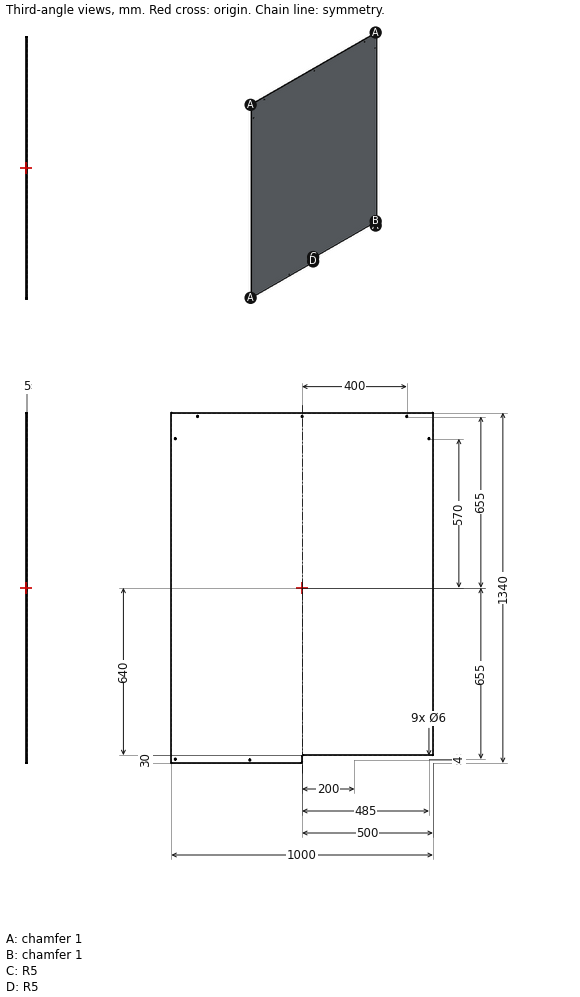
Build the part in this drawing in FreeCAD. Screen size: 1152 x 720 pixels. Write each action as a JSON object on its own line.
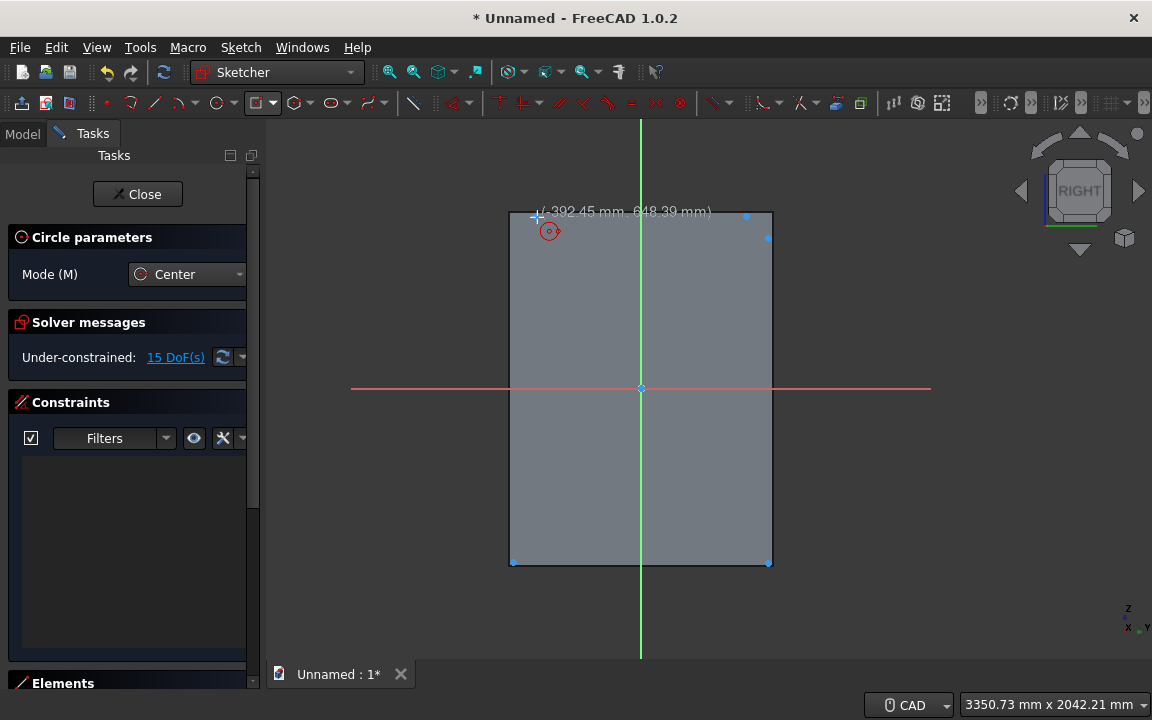
{"action": "scroll", "coordinate": [513, 238], "scroll_direction": "up", "scroll_amount": 17}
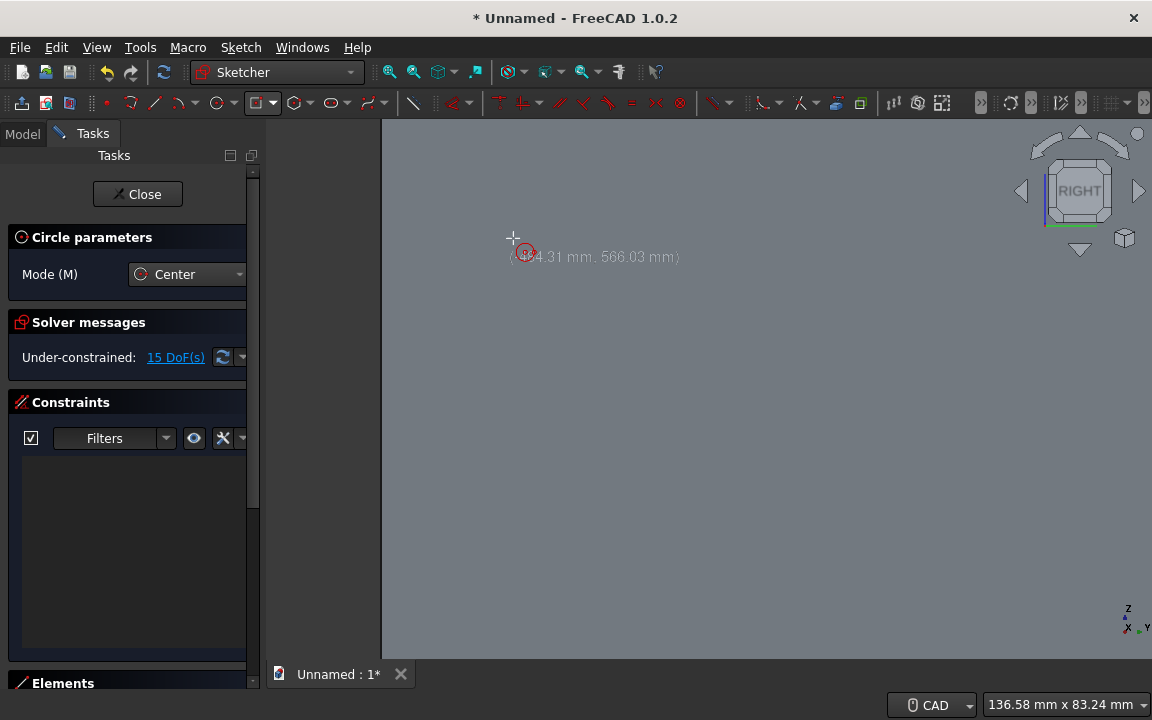
{"action": "scroll", "coordinate": [483, 203], "scroll_direction": "down", "scroll_amount": 16}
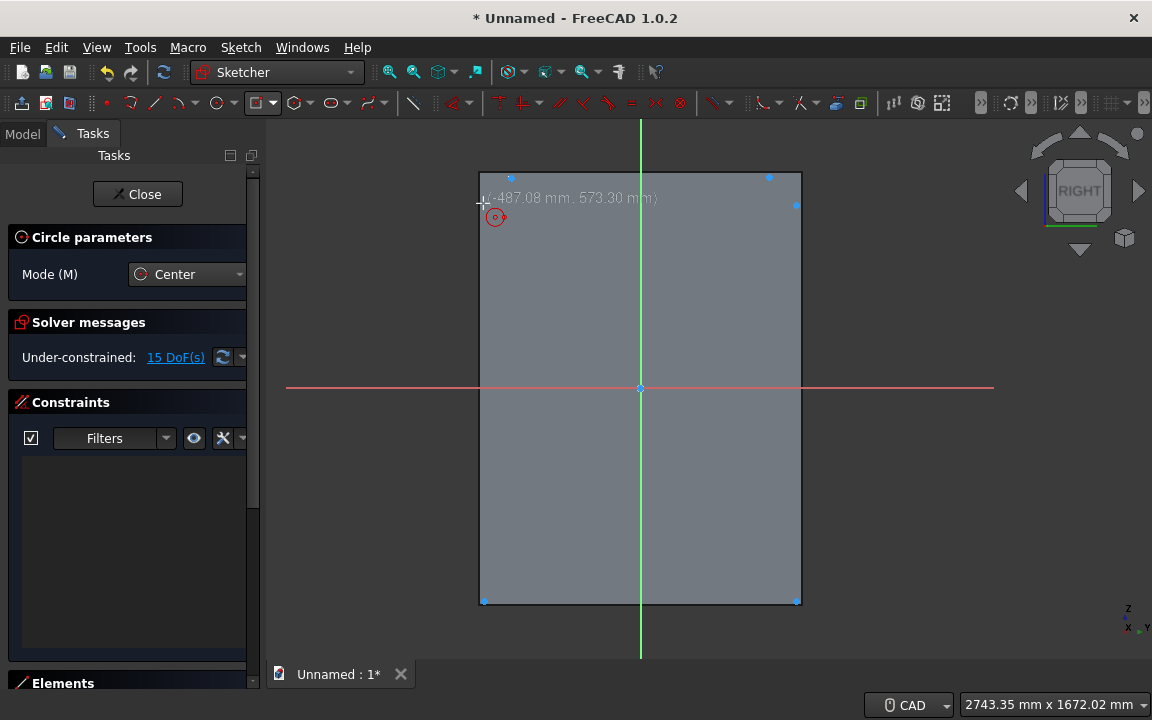
{"action": "left_click", "coordinate": [484, 204]}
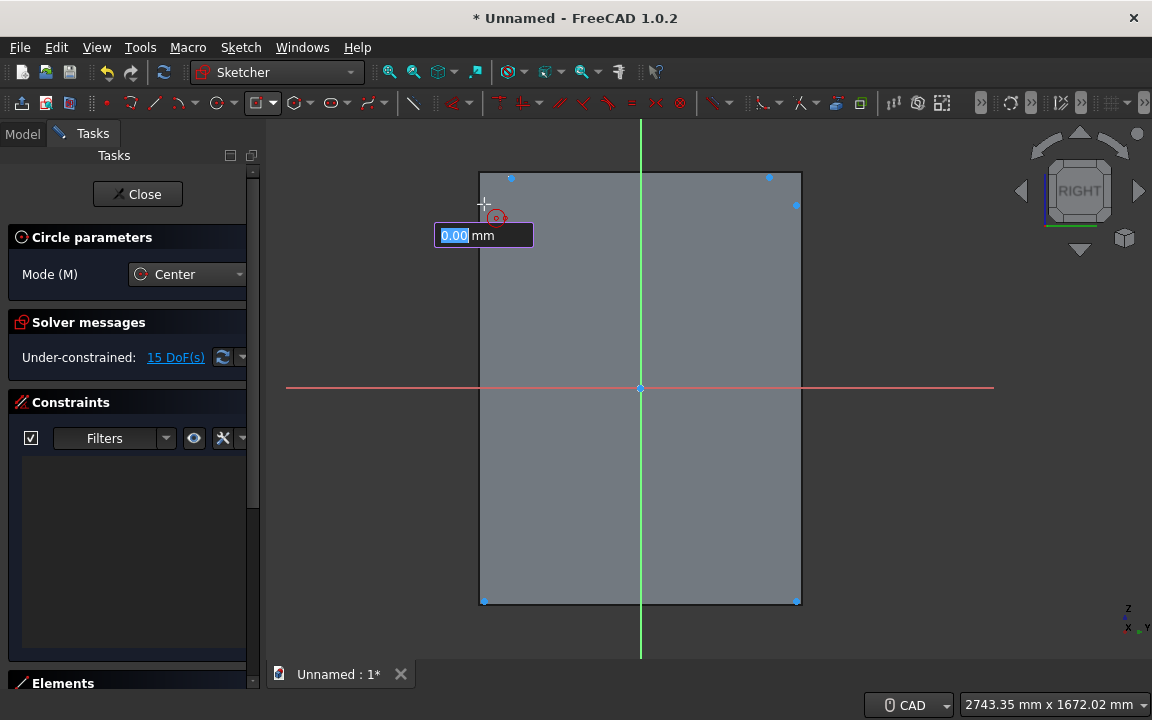
{"action": "scroll", "coordinate": [485, 204], "scroll_direction": "up", "scroll_amount": 14}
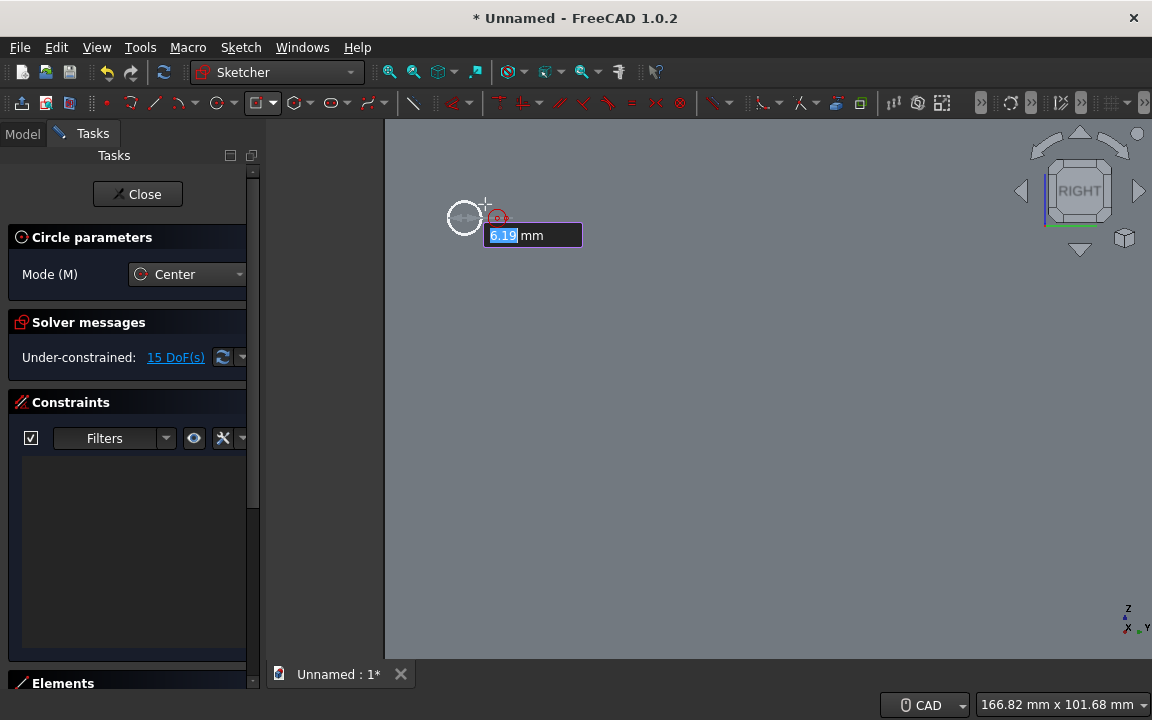
{"action": "left_click", "coordinate": [474, 194]}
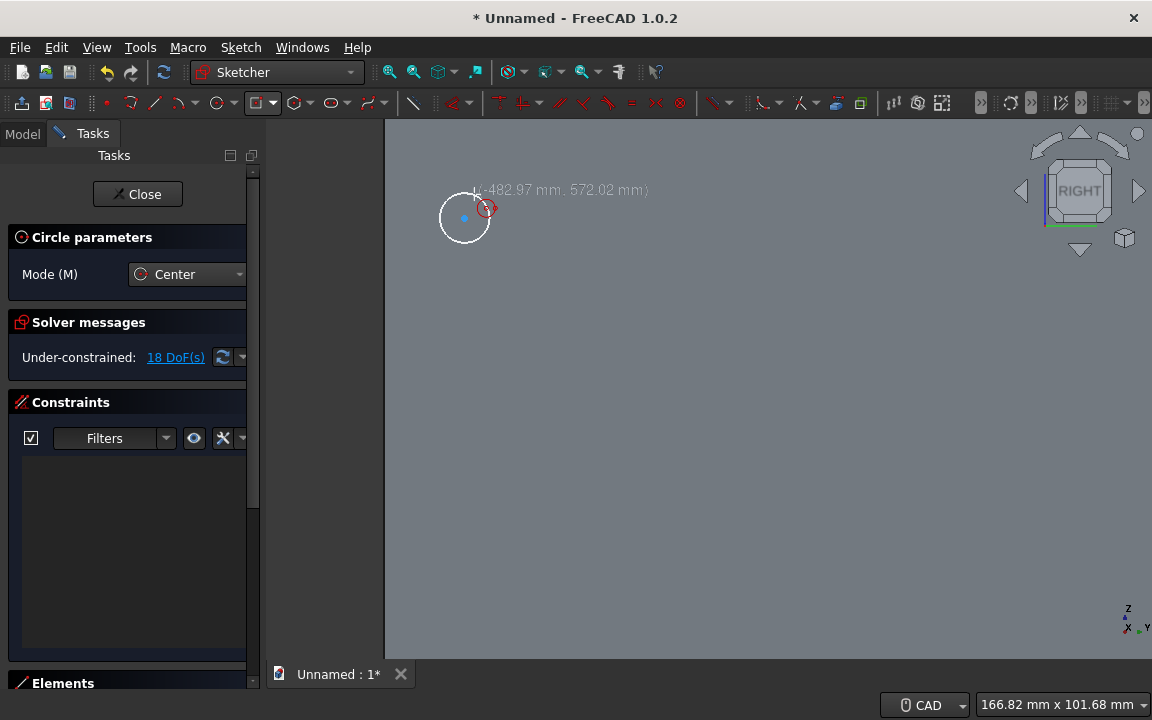
{"action": "scroll", "coordinate": [515, 239], "scroll_direction": "down", "scroll_amount": 15}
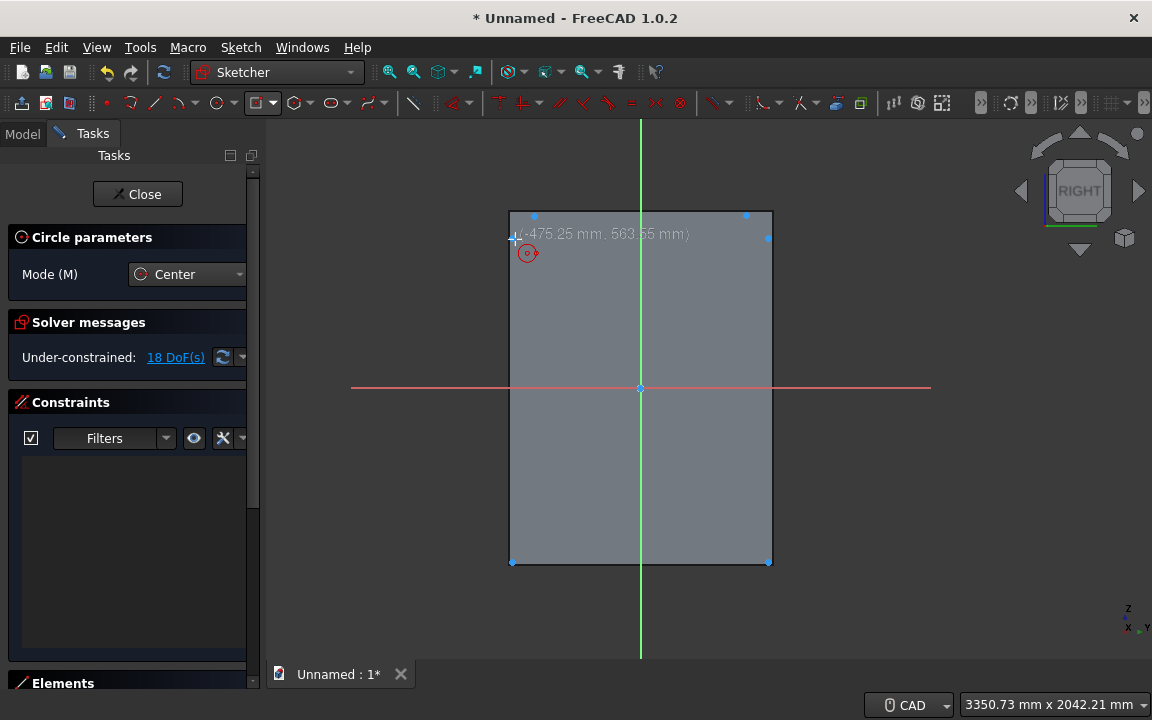
{"action": "scroll", "coordinate": [641, 215], "scroll_direction": "up", "scroll_amount": 17}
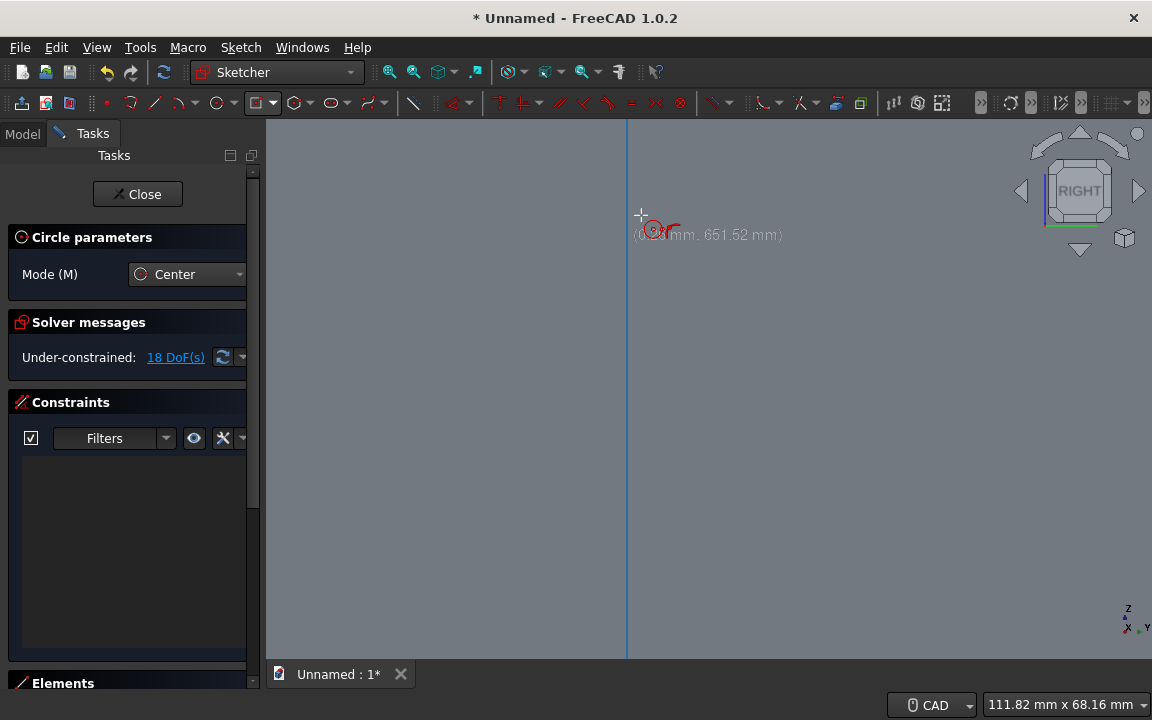
{"action": "scroll", "coordinate": [641, 175], "scroll_direction": "down", "scroll_amount": 16}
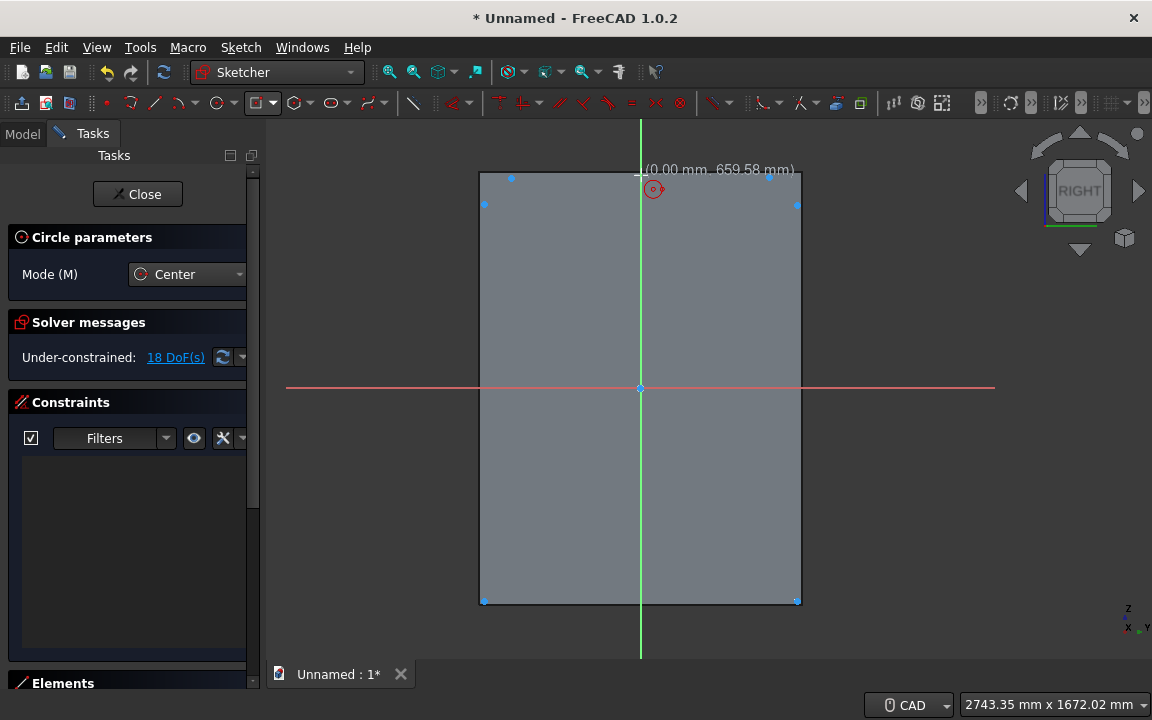
{"action": "left_click", "coordinate": [641, 177]}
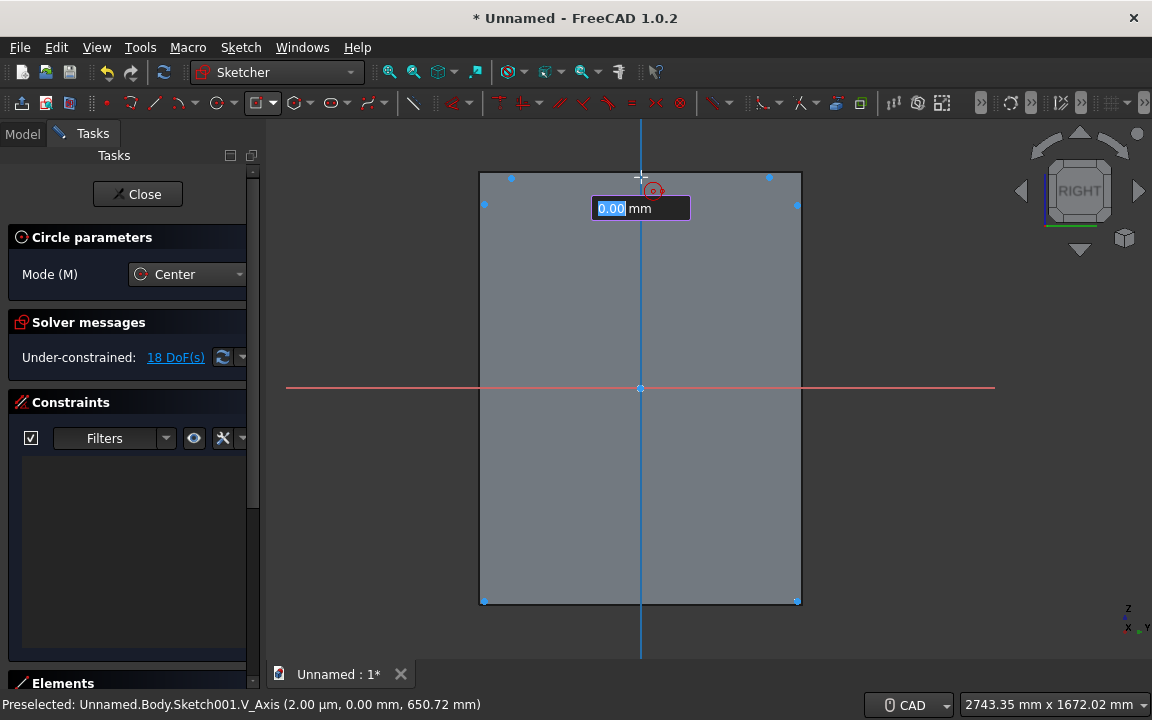
{"action": "scroll", "coordinate": [642, 176], "scroll_direction": "up", "scroll_amount": 15}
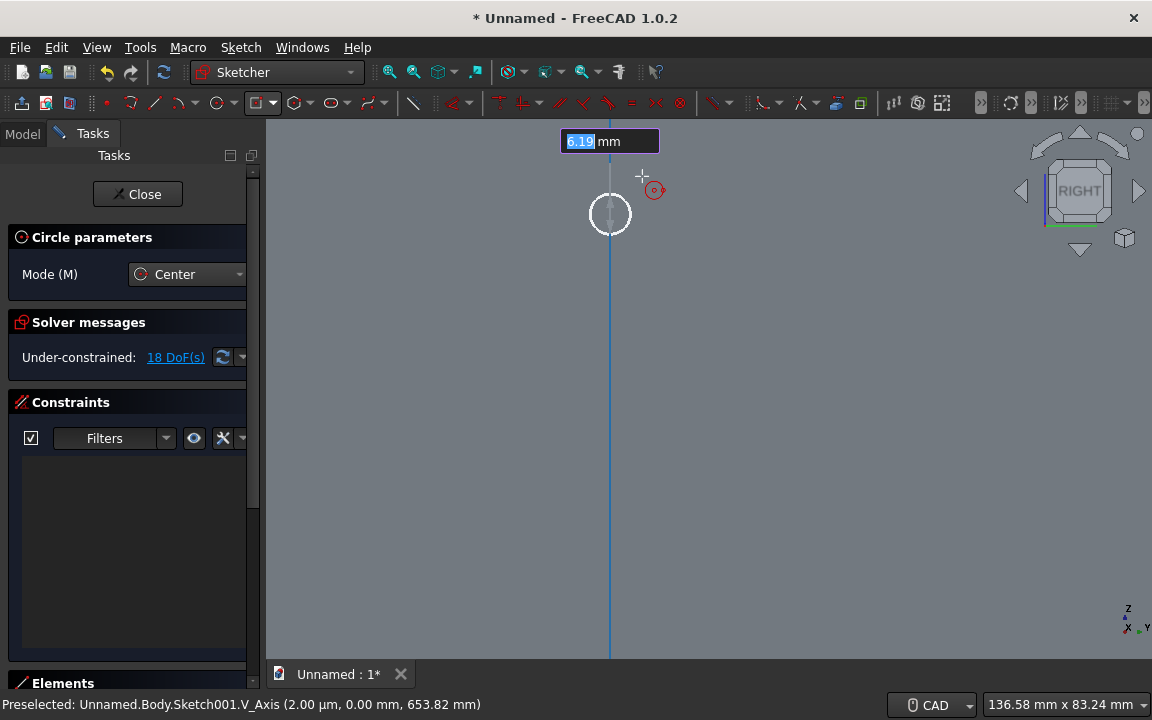
{"action": "left_click", "coordinate": [629, 180]}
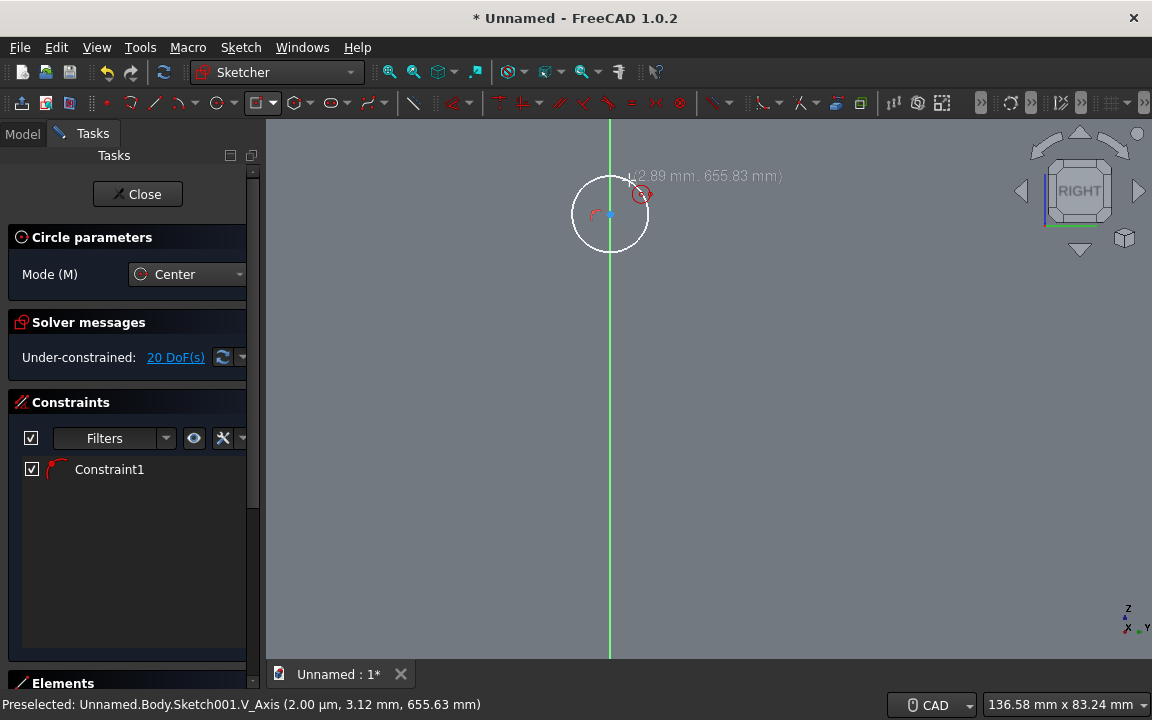
{"action": "scroll", "coordinate": [642, 176], "scroll_direction": "down", "scroll_amount": 15}